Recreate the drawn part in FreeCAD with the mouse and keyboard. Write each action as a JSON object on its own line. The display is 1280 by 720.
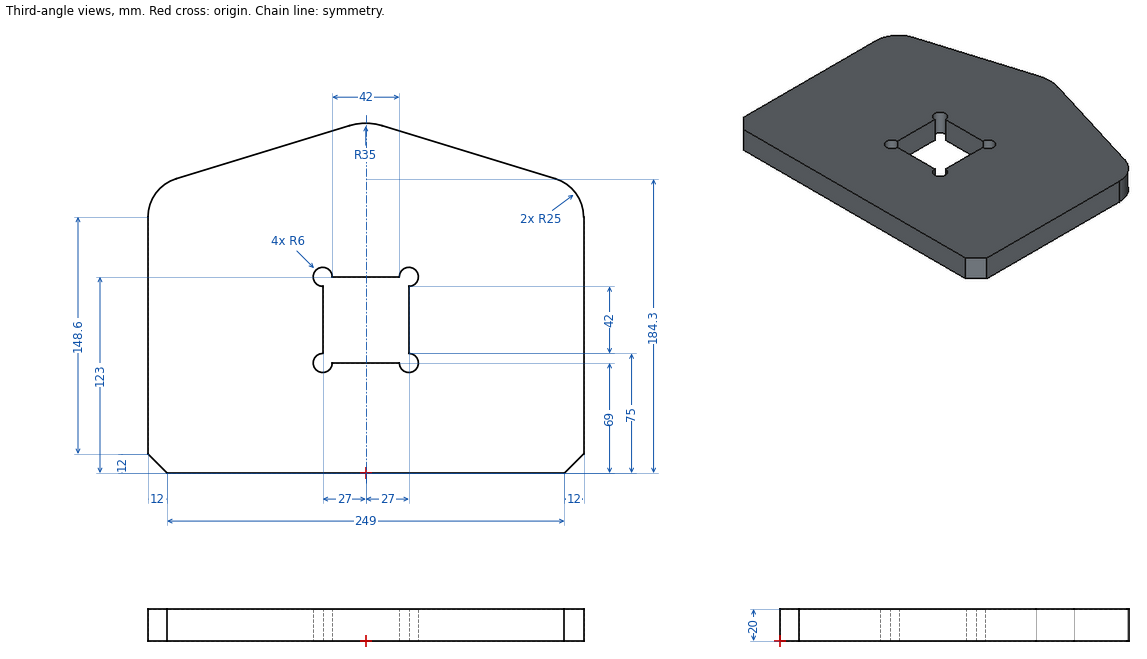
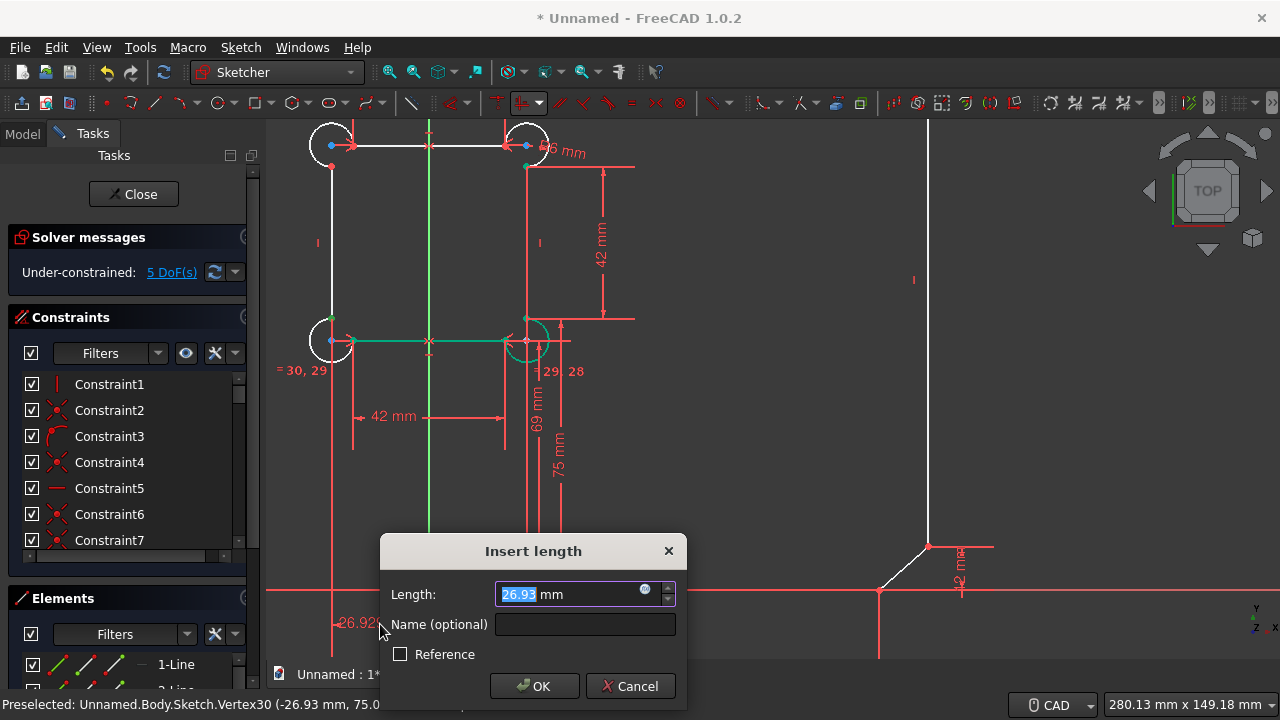
{"action": "type", "text": "27"}
{"action": "key", "text": "Return"}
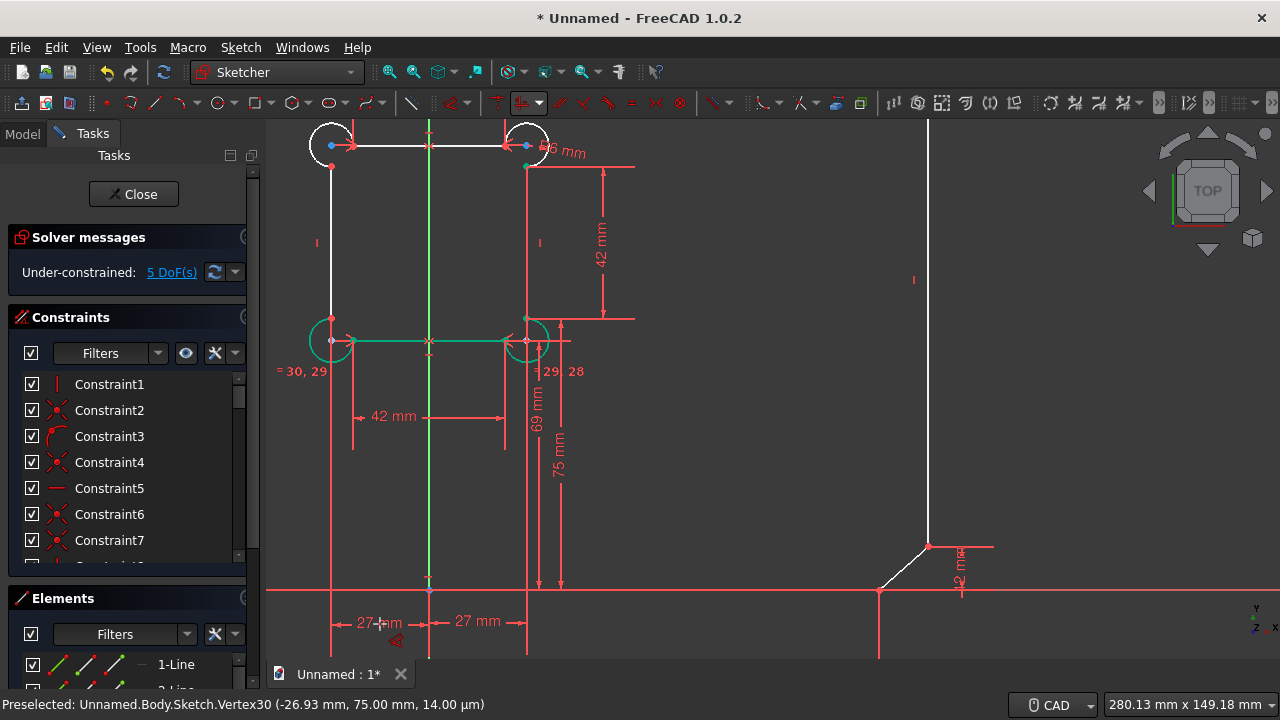
{"action": "scroll", "coordinate": [929, 549], "scroll_direction": "down", "scroll_amount": 4}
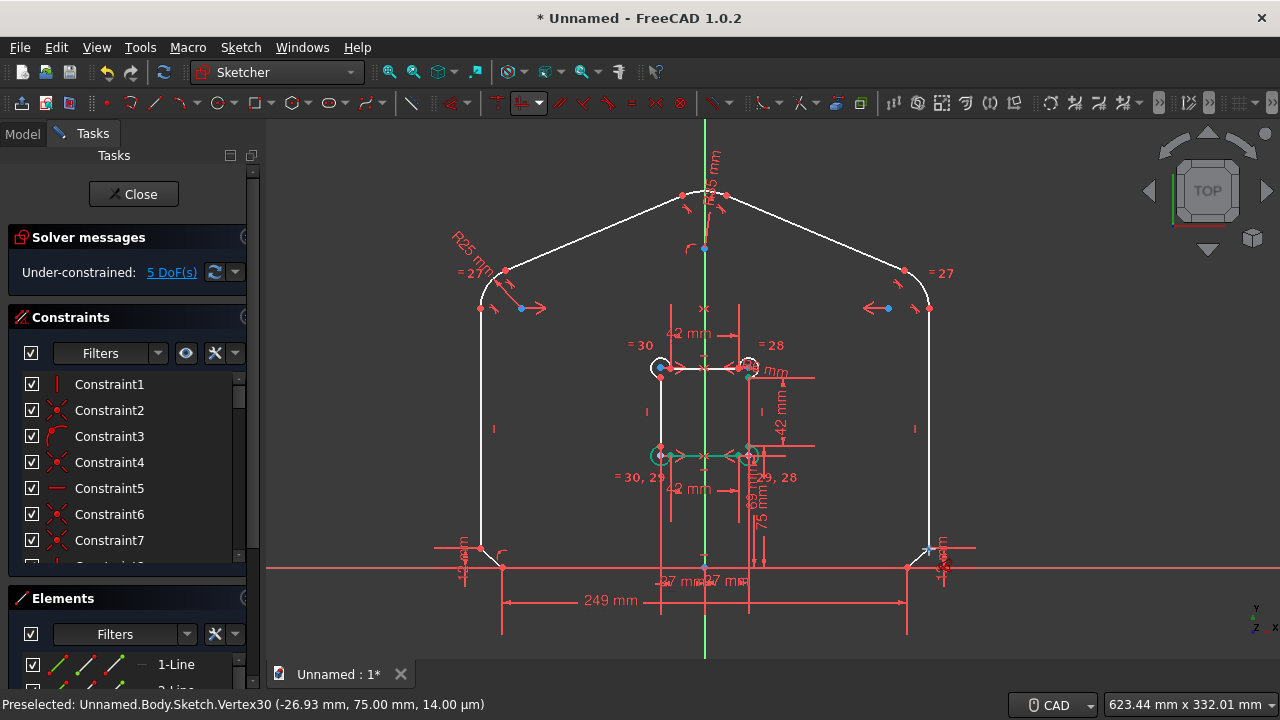
{"action": "scroll", "coordinate": [487, 554], "scroll_direction": "up", "scroll_amount": 4}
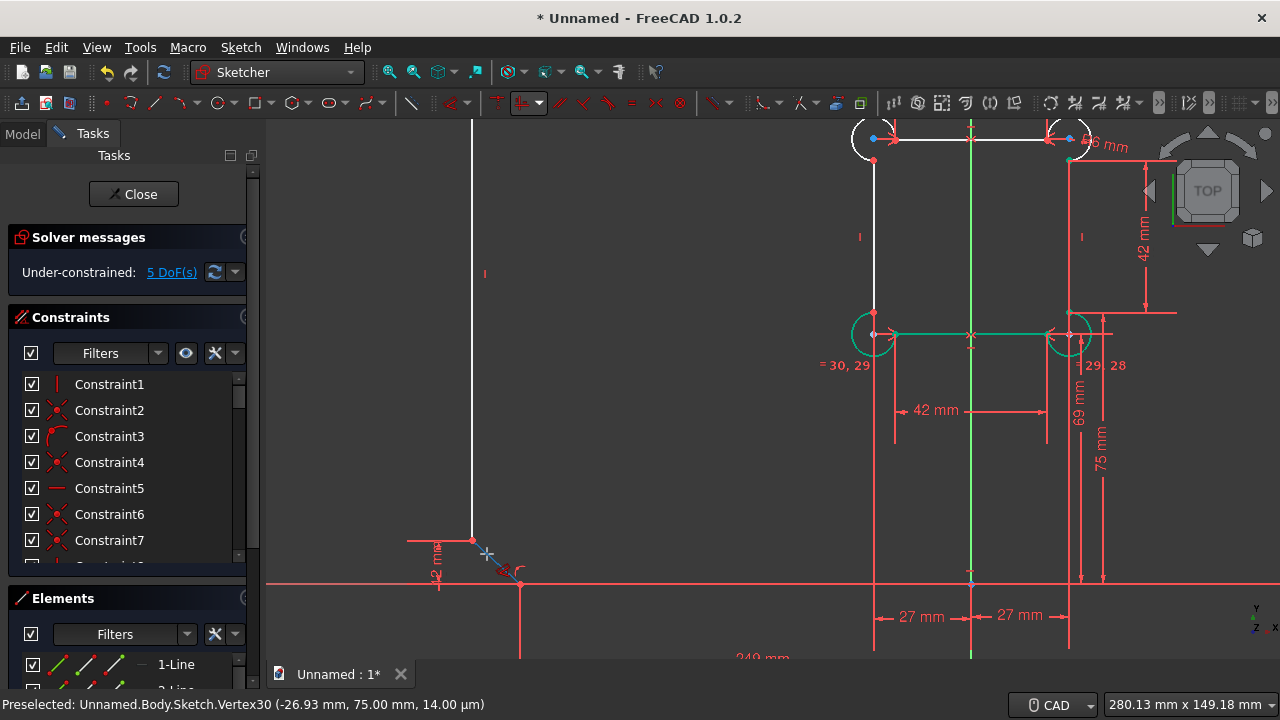
{"action": "left_click", "coordinate": [487, 554]}
{"action": "left_click", "coordinate": [496, 618]}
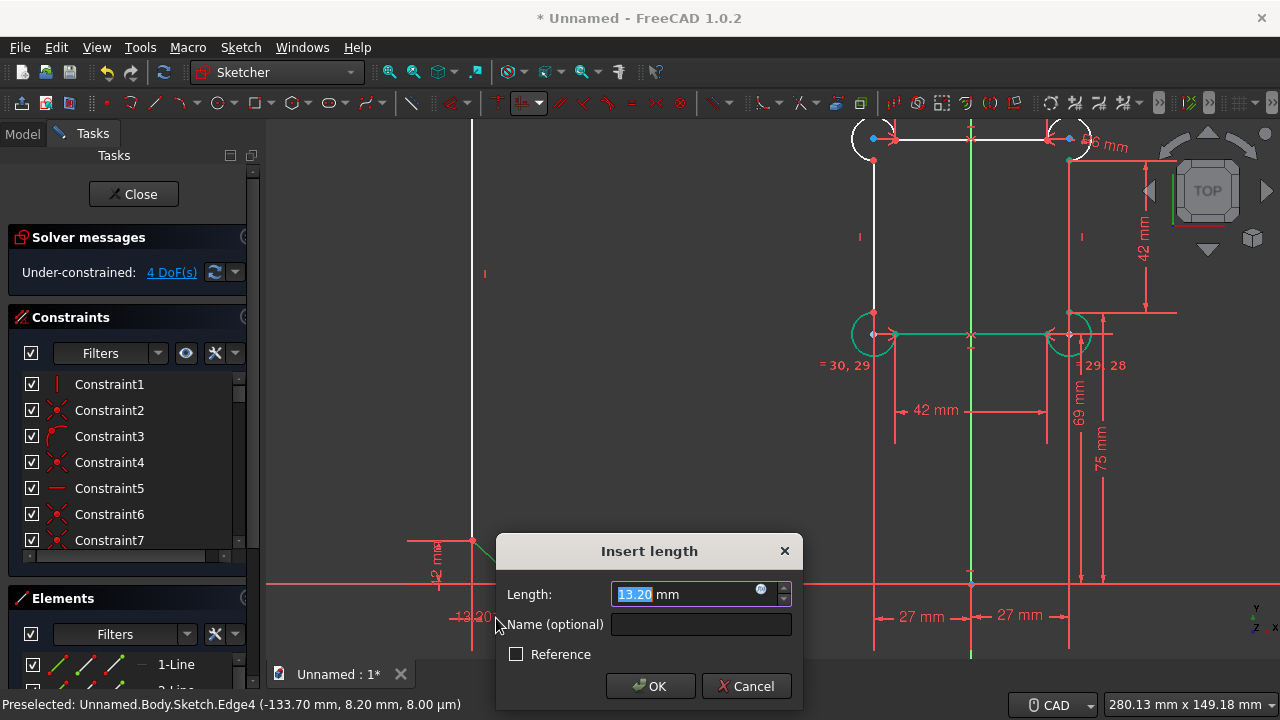
{"action": "type", "text": "12"}
{"action": "key", "text": "Return"}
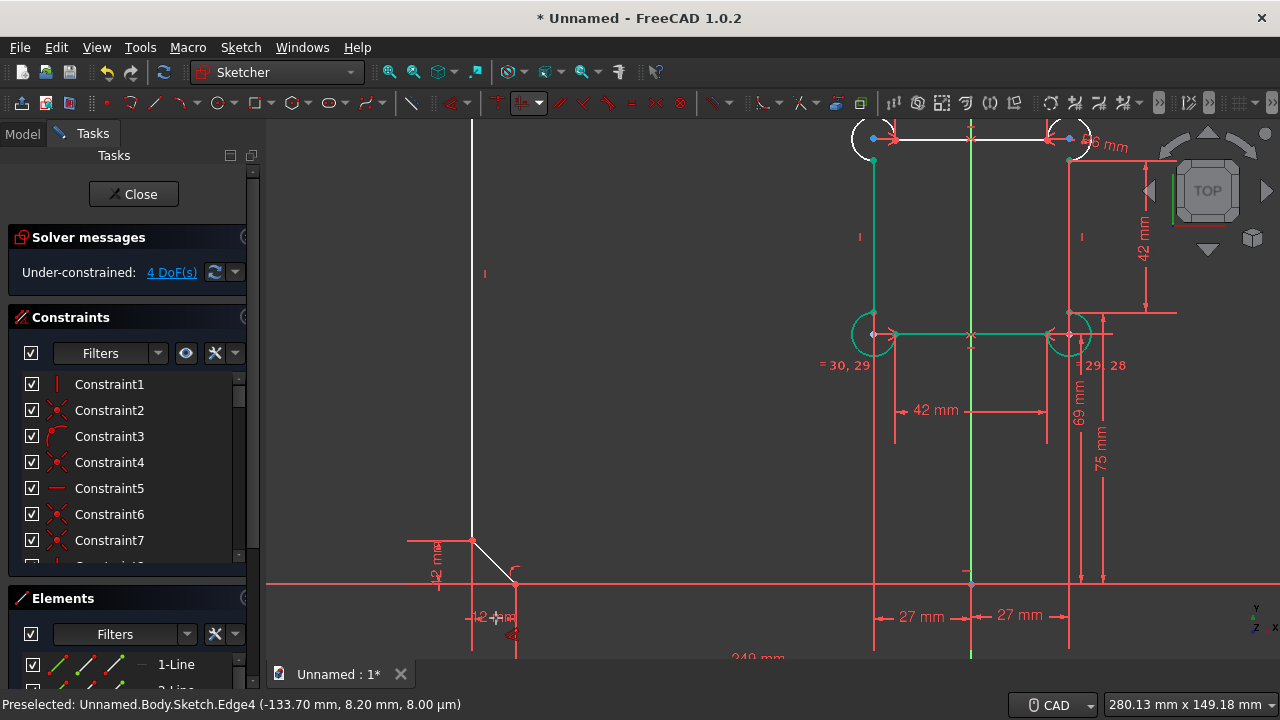
{"action": "scroll", "coordinate": [487, 554], "scroll_direction": "down", "scroll_amount": 4}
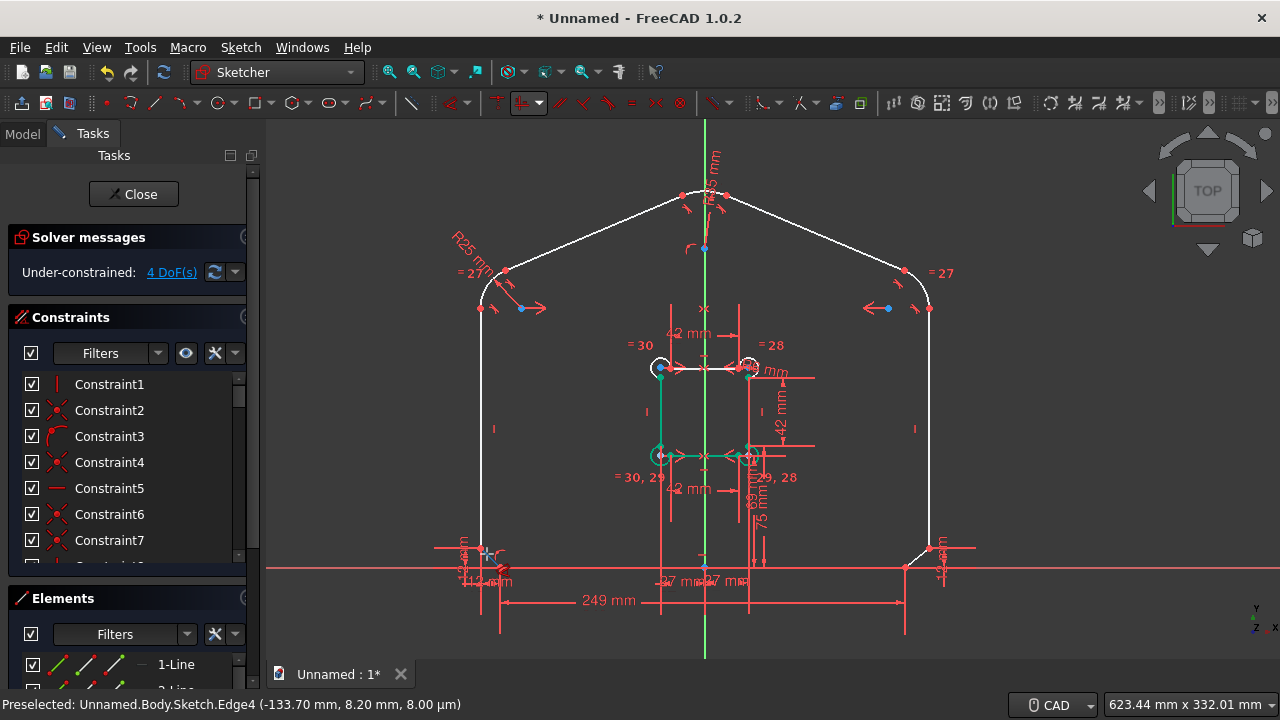
{"action": "scroll", "coordinate": [912, 562], "scroll_direction": "up", "scroll_amount": 5}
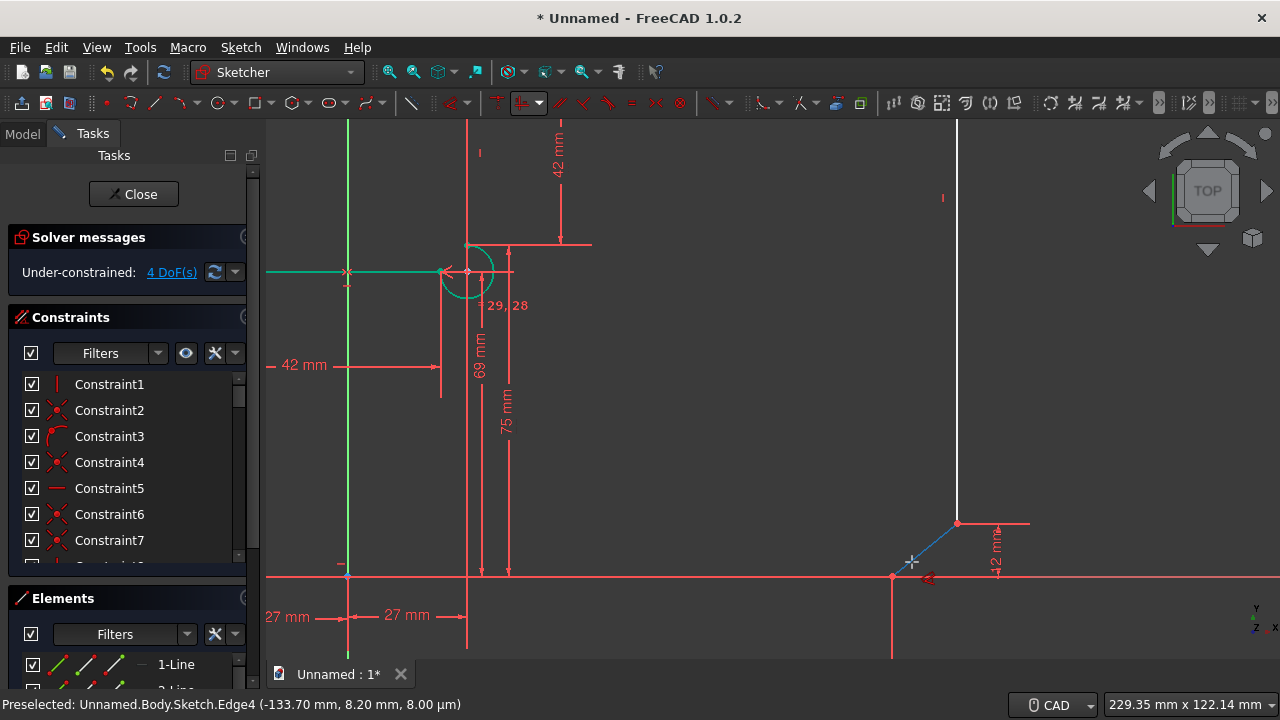
{"action": "left_click", "coordinate": [912, 561]}
{"action": "left_click", "coordinate": [925, 611]}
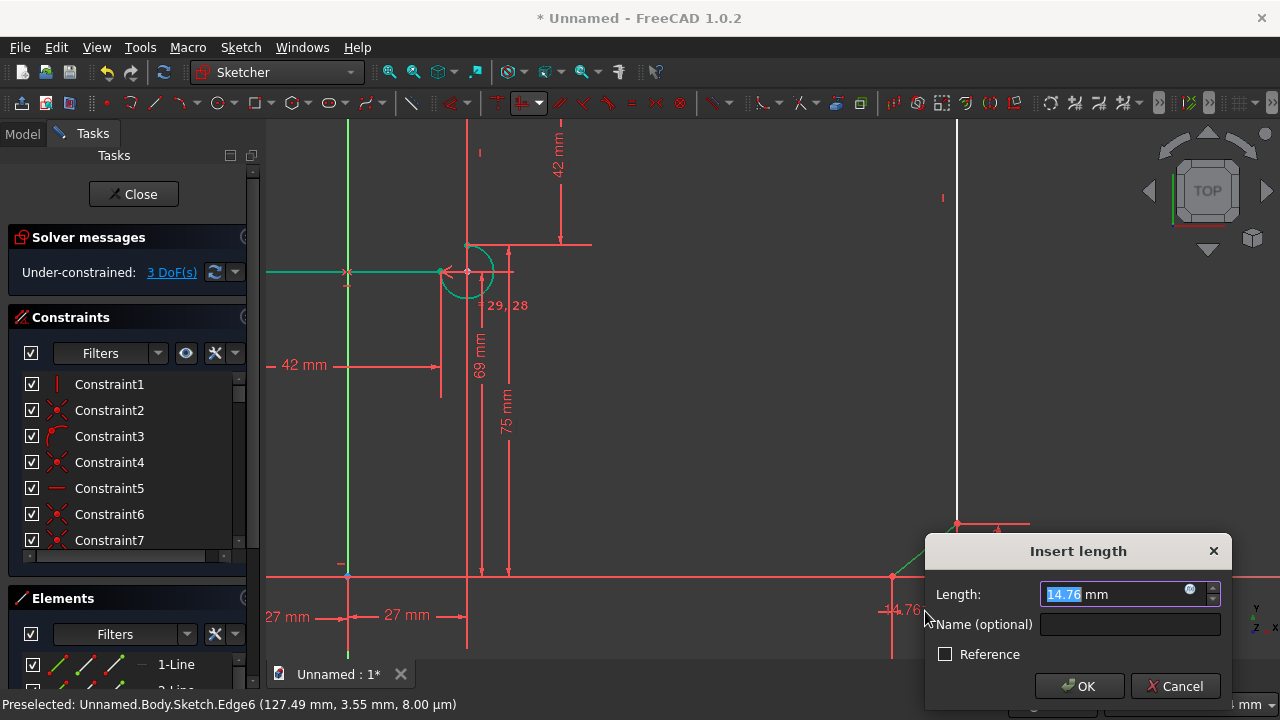
{"action": "type", "text": "12"}
{"action": "key", "text": "Return"}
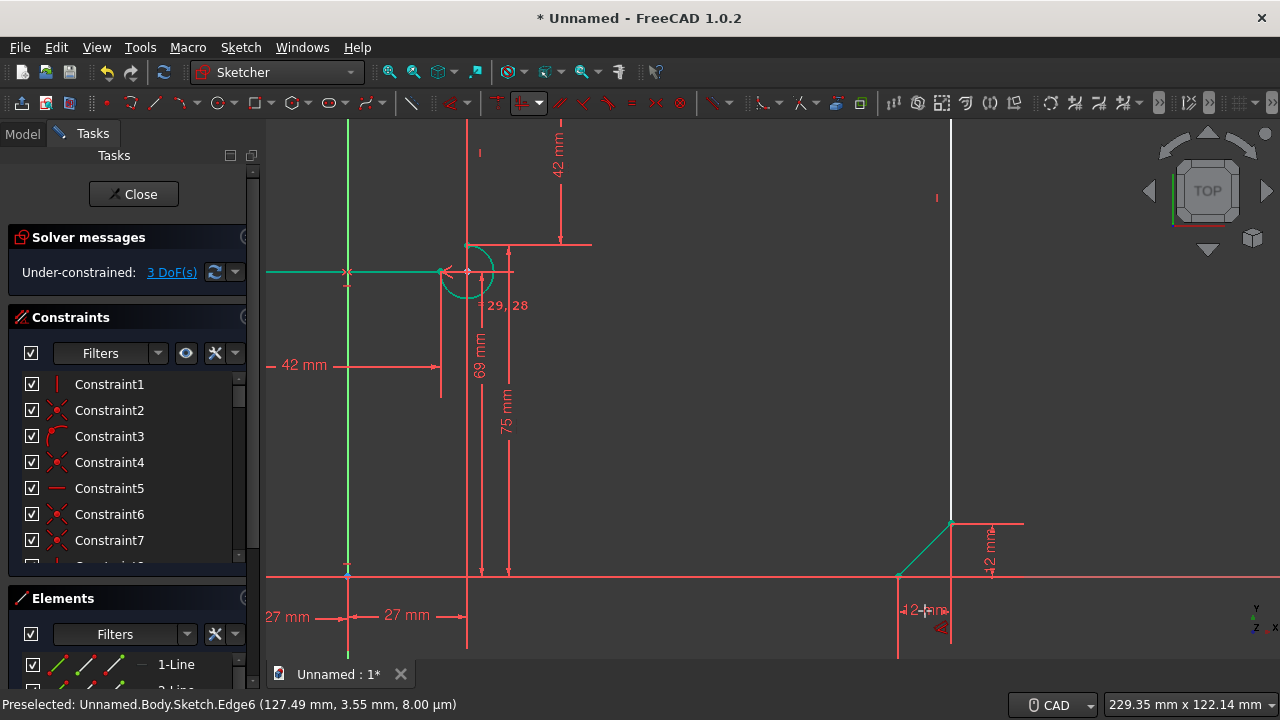
{"action": "scroll", "coordinate": [912, 562], "scroll_direction": "down", "scroll_amount": 5}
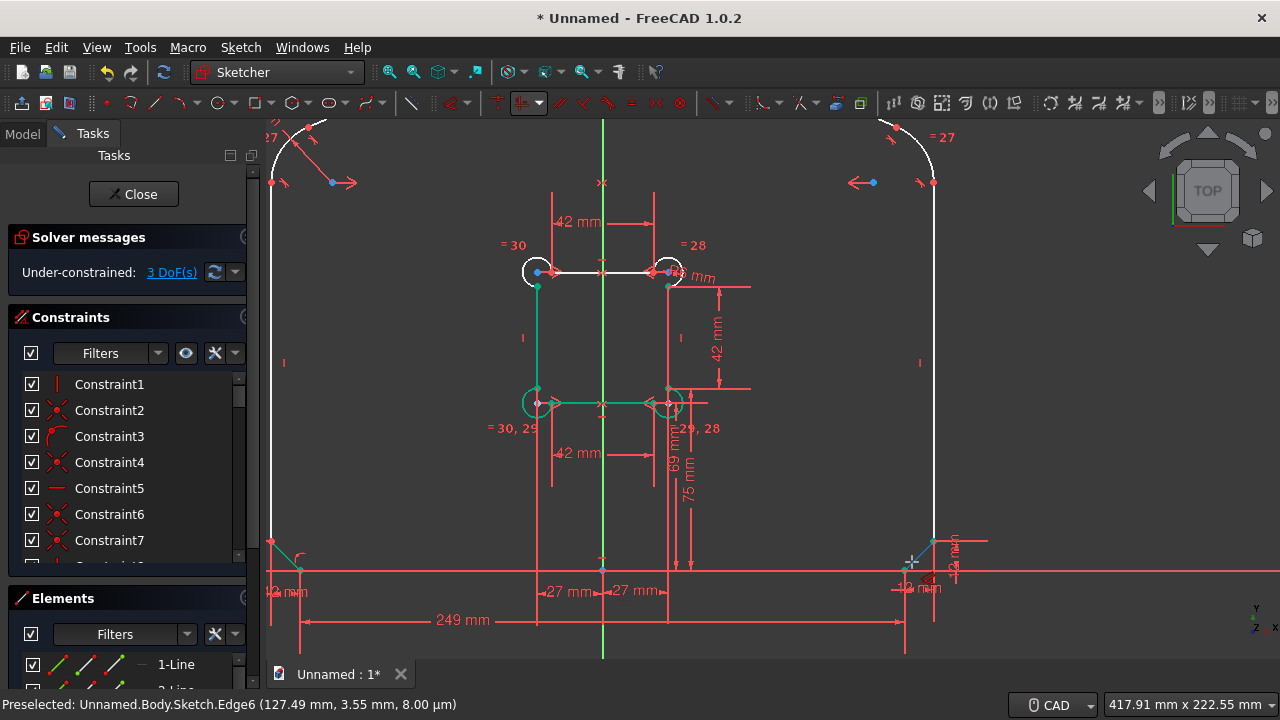
{"action": "scroll", "coordinate": [671, 369], "scroll_direction": "up", "scroll_amount": 2}